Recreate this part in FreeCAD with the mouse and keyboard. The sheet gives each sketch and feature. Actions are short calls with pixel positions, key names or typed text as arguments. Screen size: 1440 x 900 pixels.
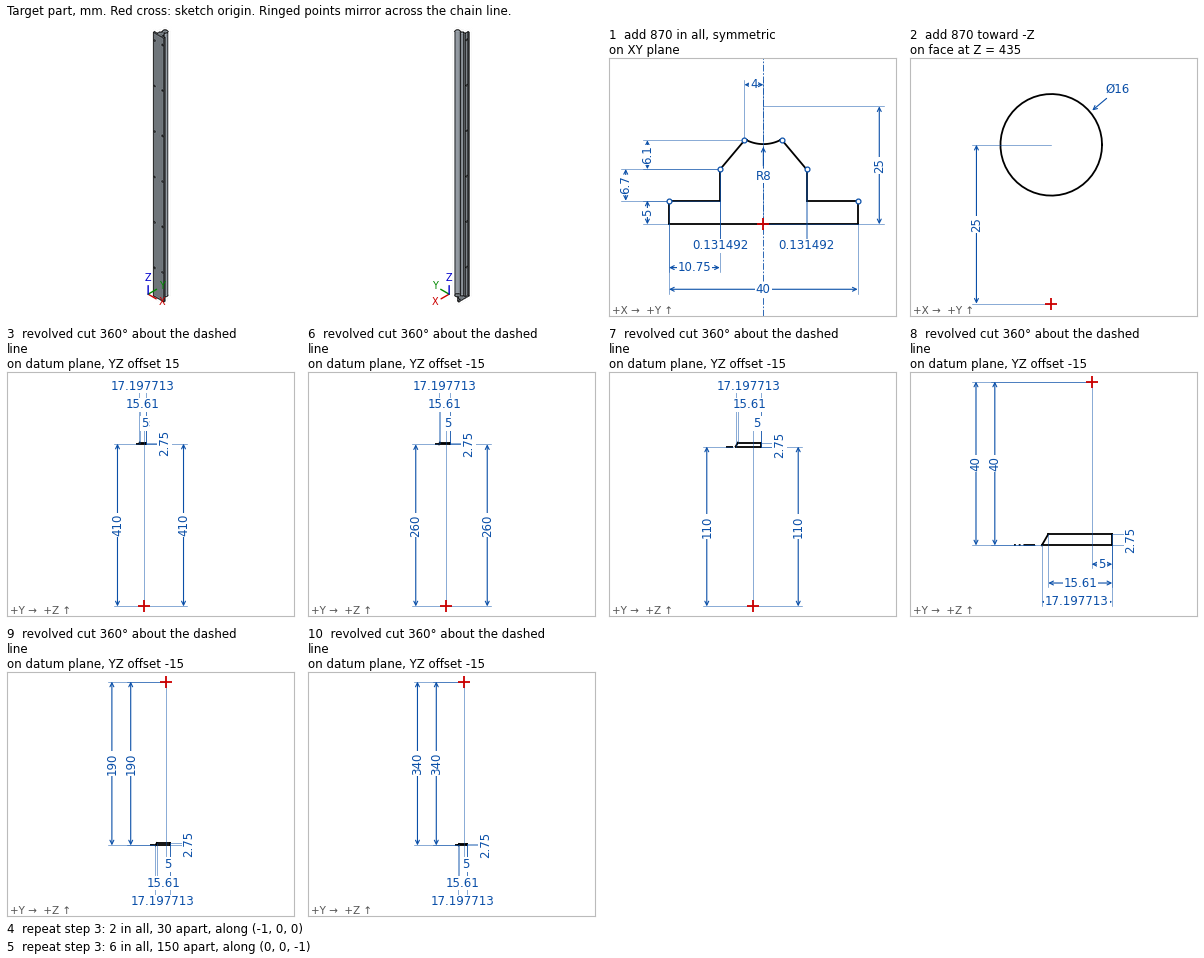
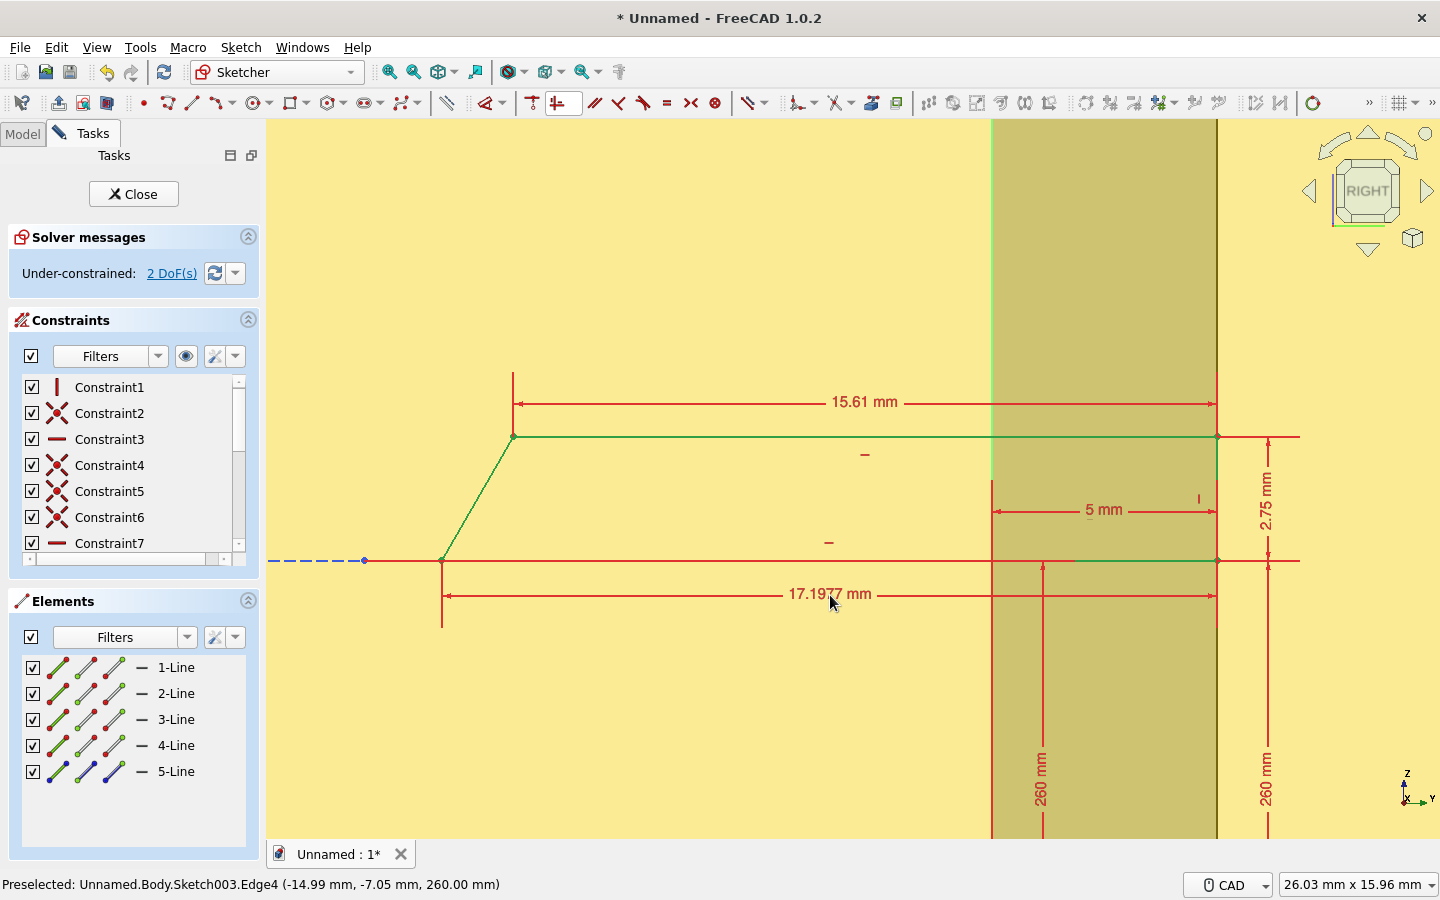
click(134, 194)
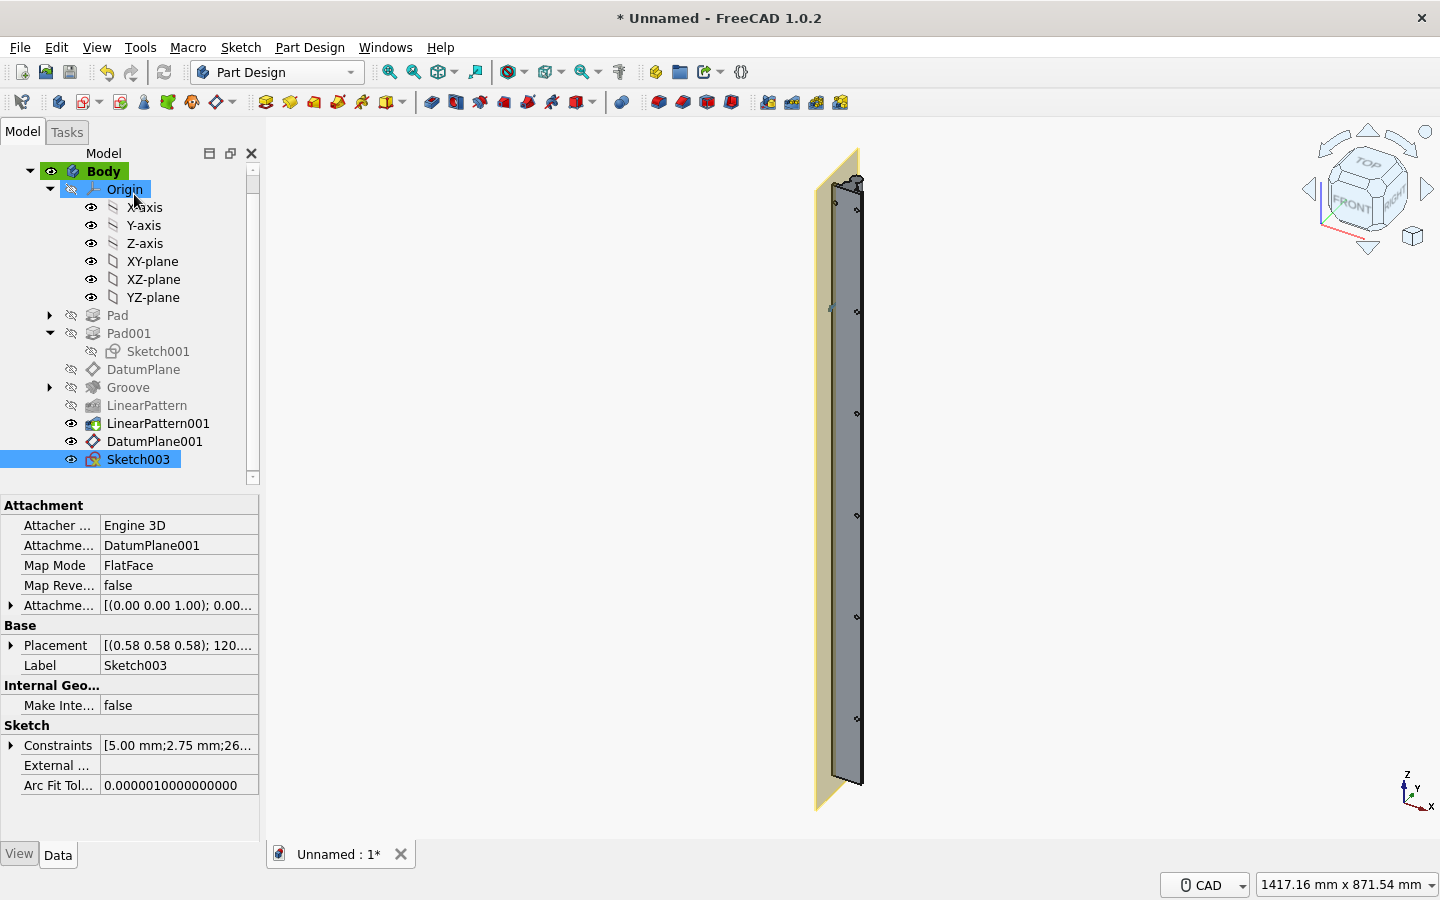
click(480, 102)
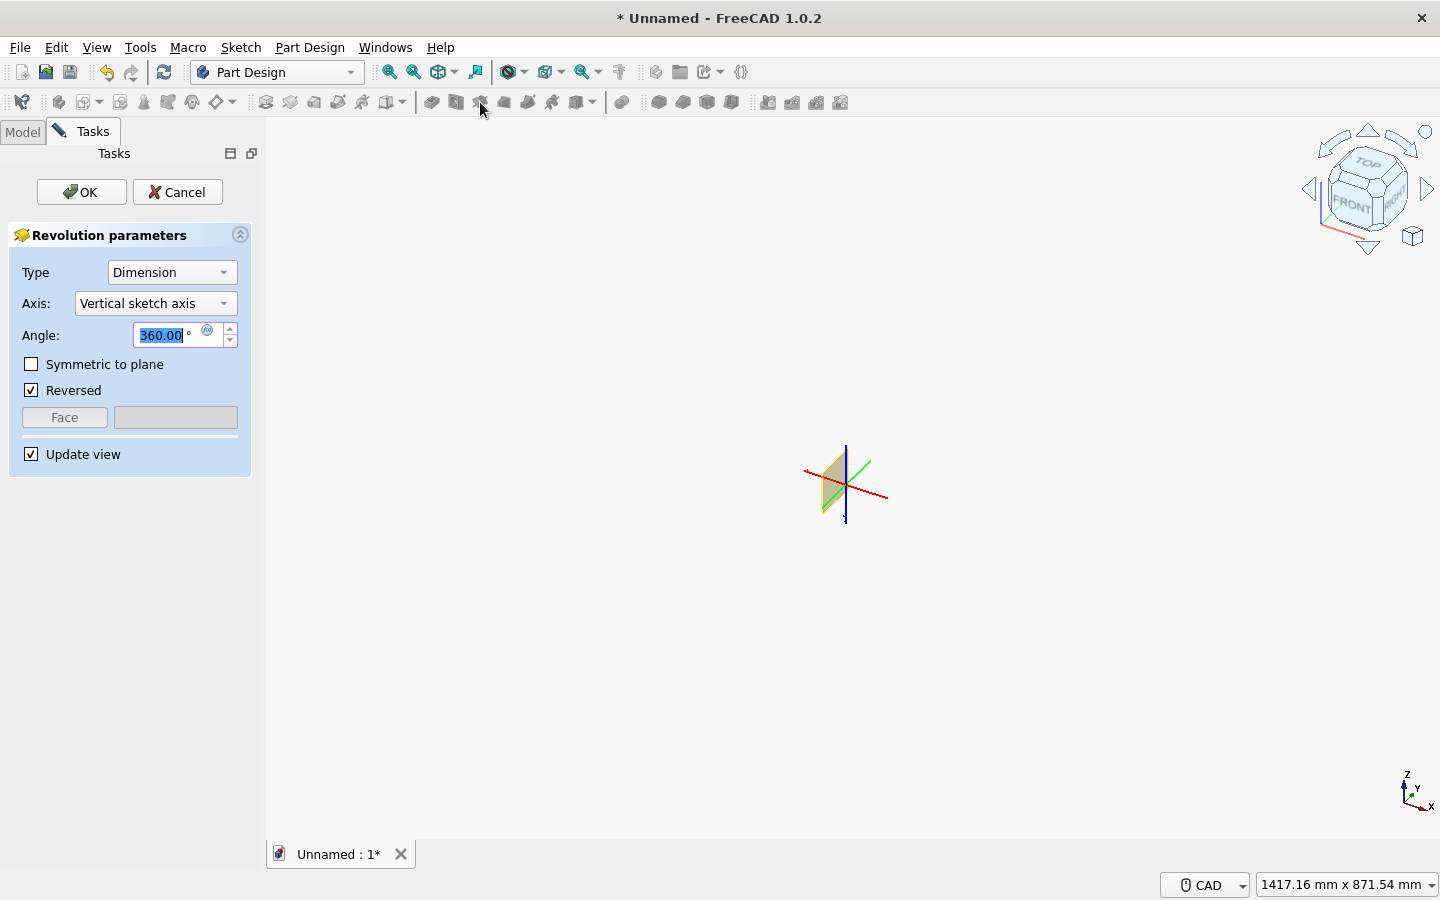
click(156, 304)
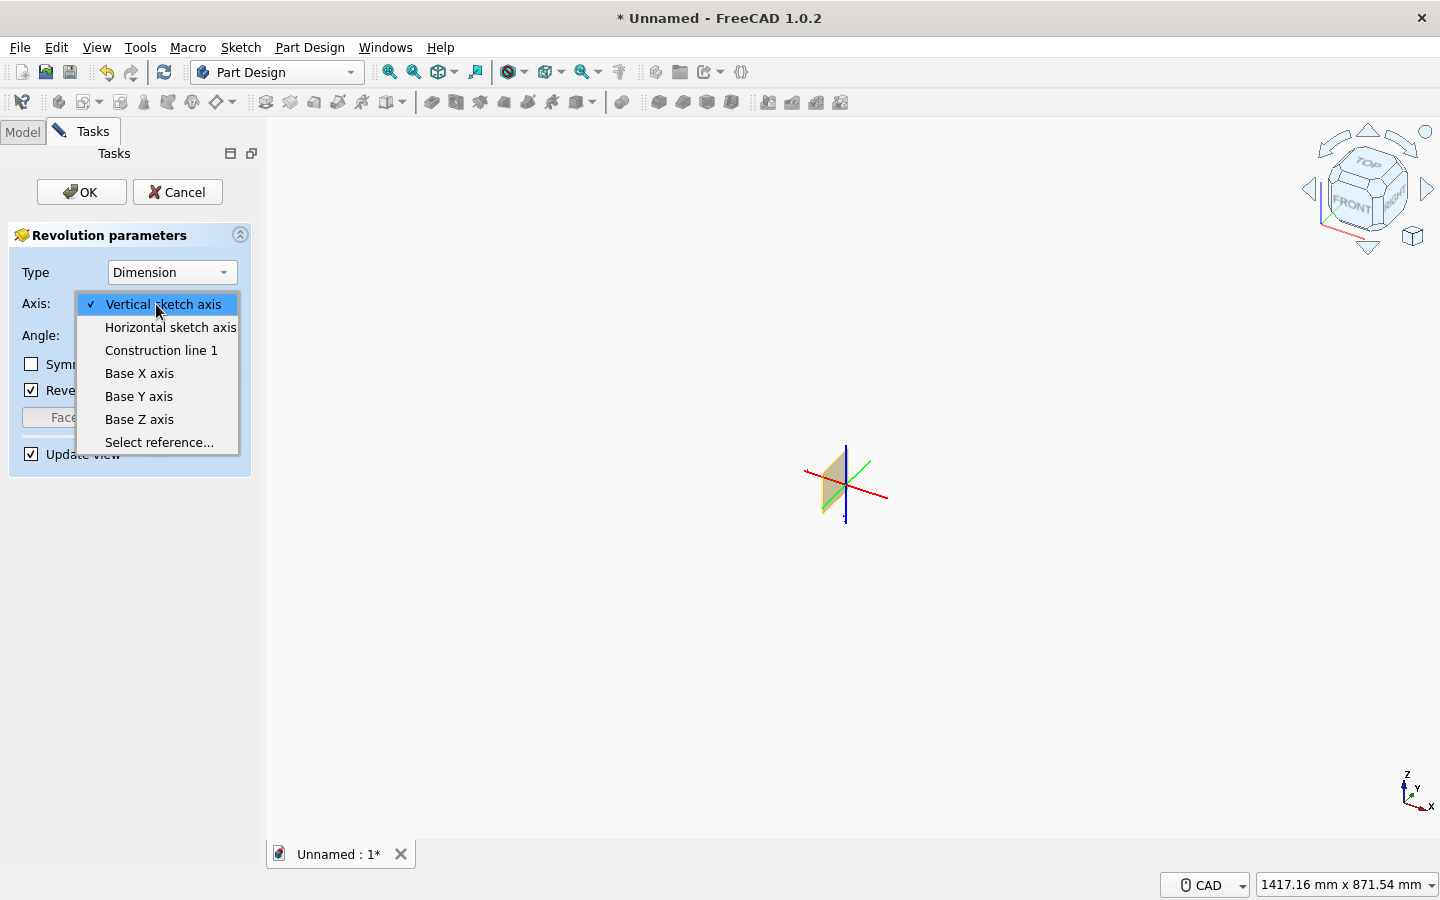
click(156, 350)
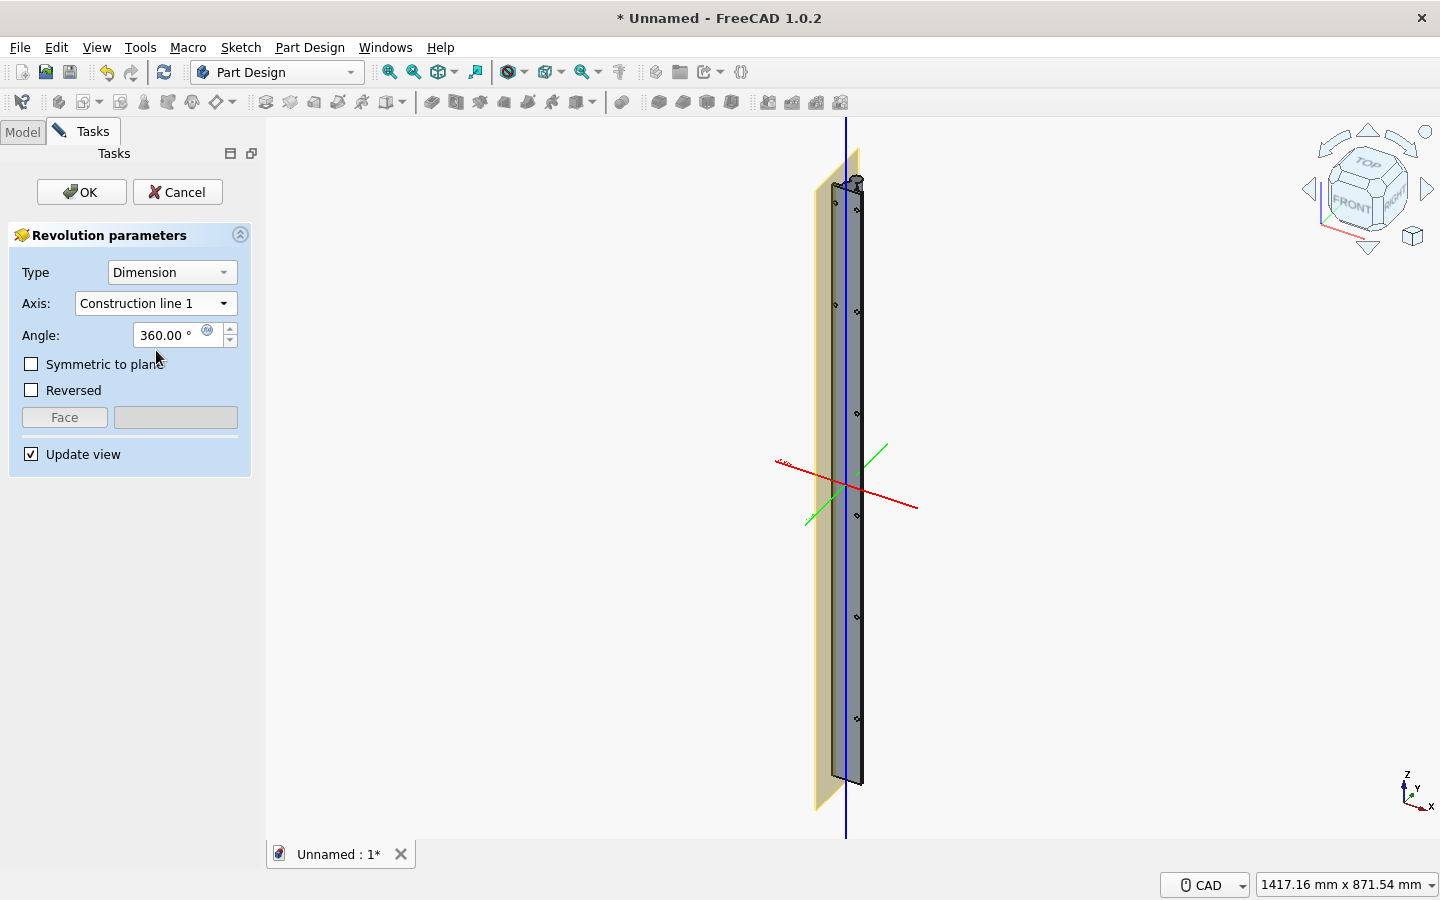
click(82, 192)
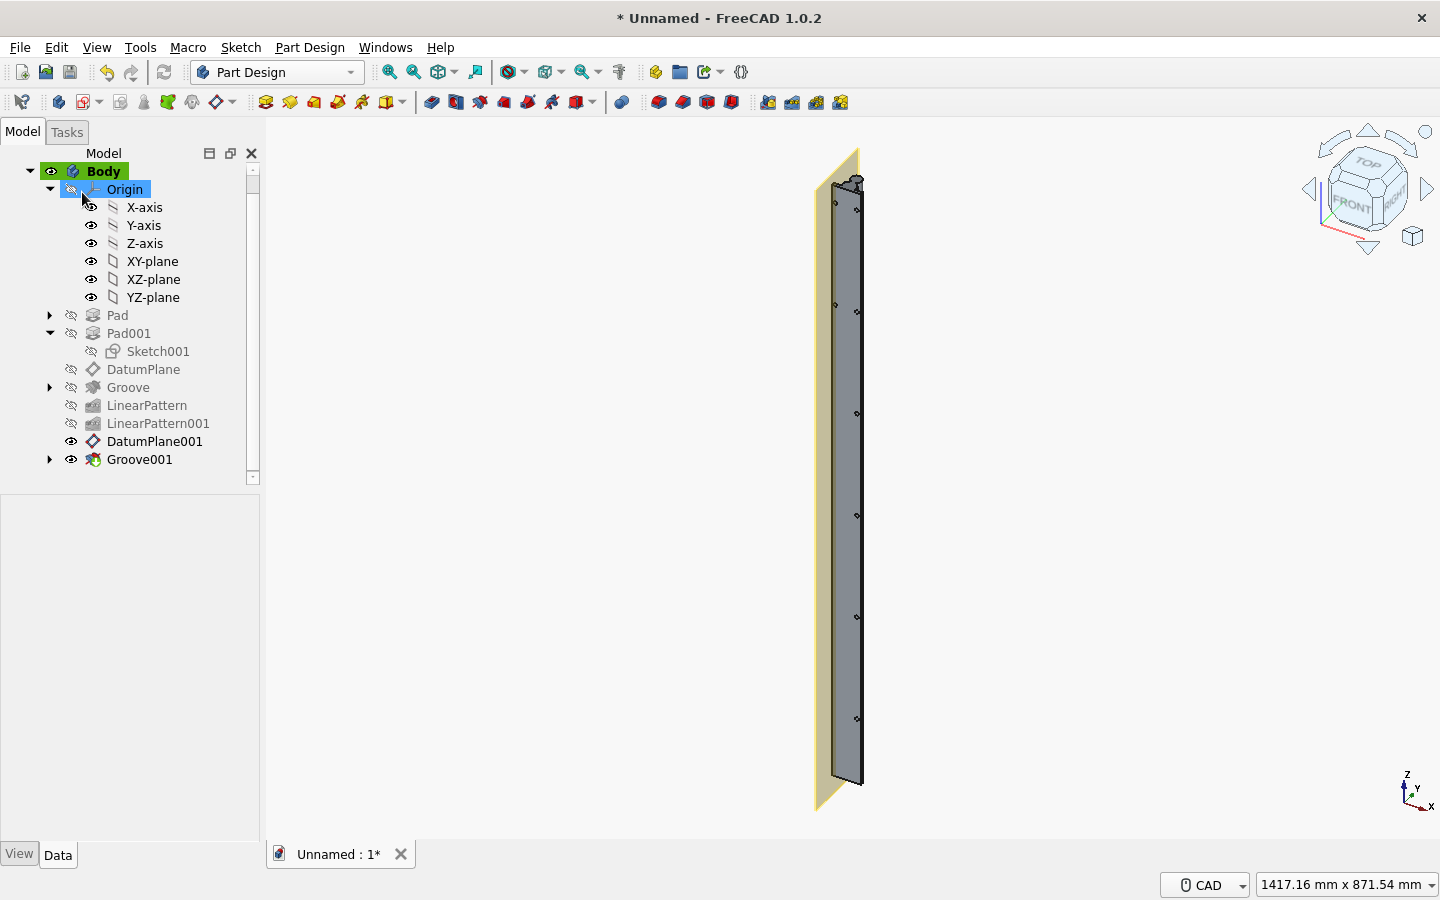
click(116, 441)
key(space)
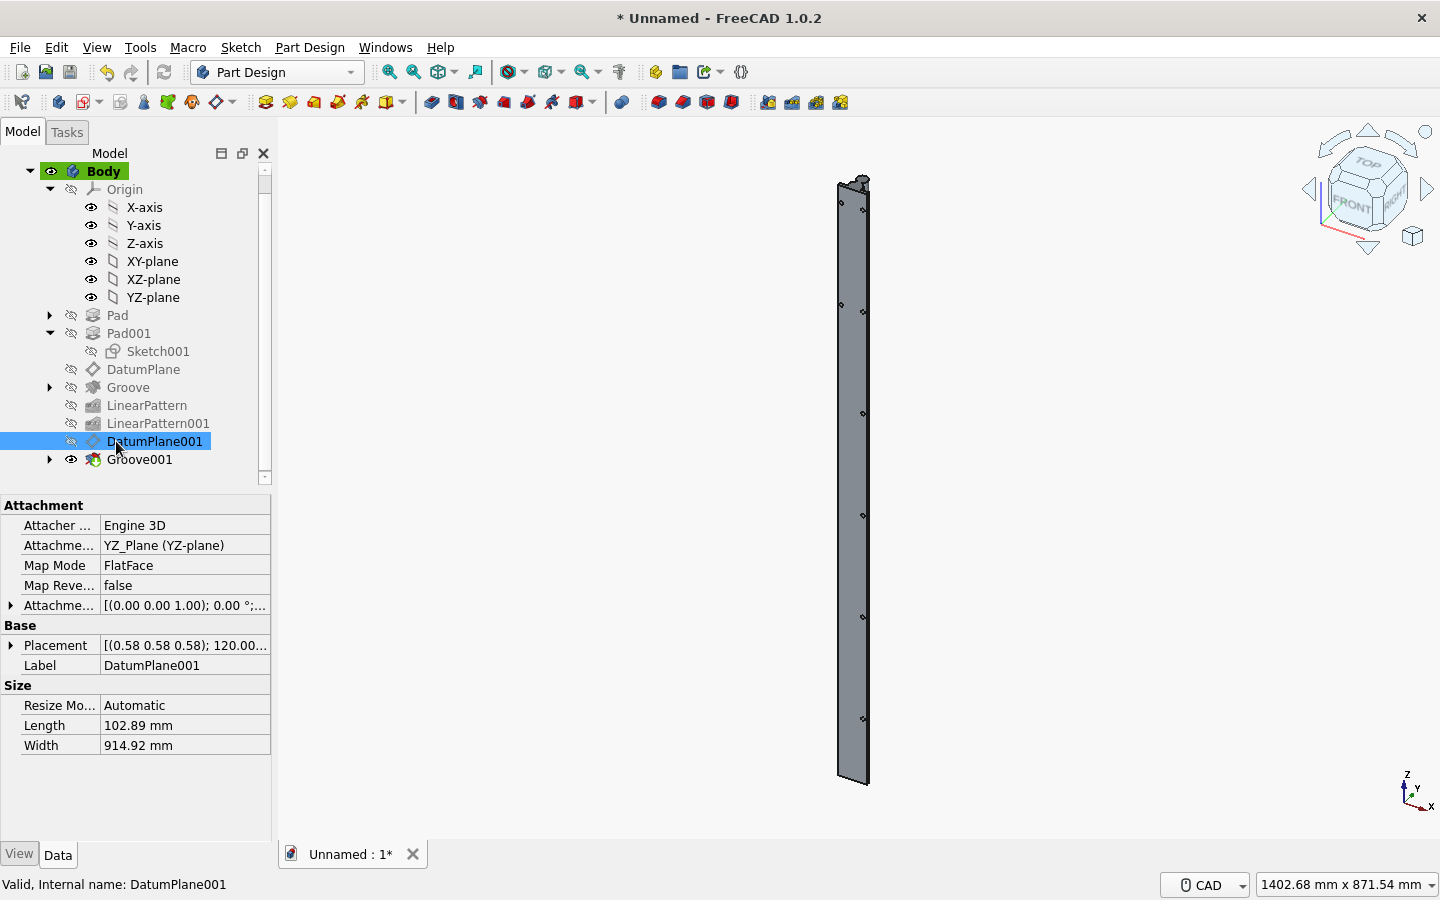
click(136, 297)